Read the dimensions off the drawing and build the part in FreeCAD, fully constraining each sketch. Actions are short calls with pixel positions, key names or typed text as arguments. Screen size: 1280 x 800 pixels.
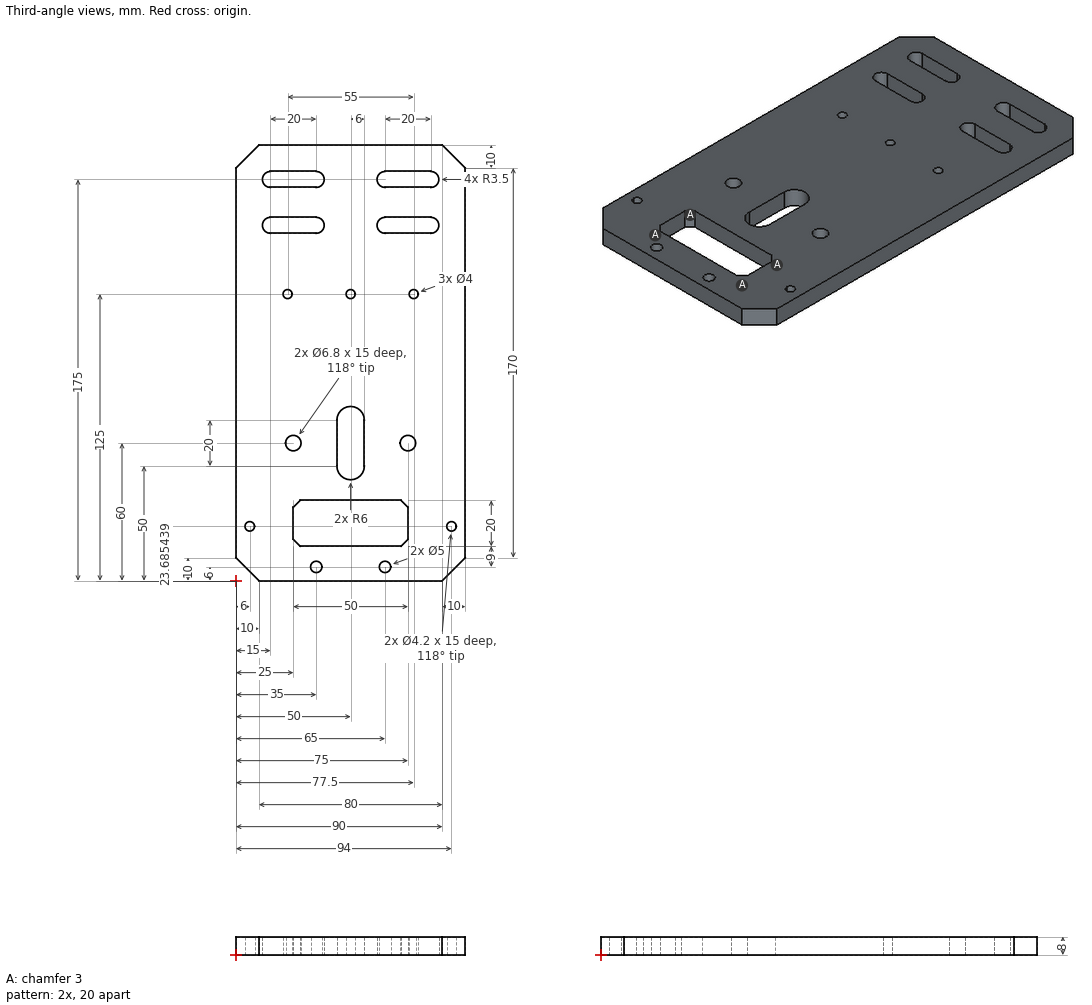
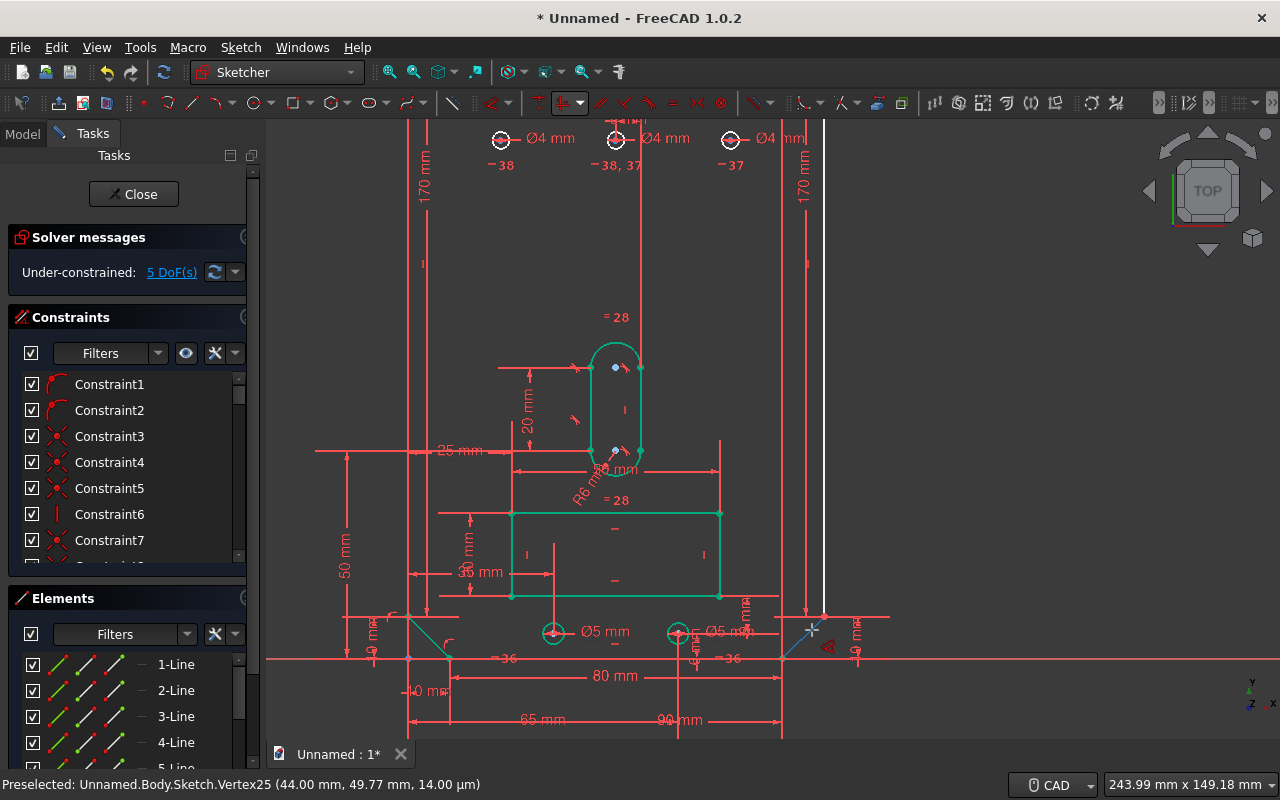
click(812, 629)
click(803, 693)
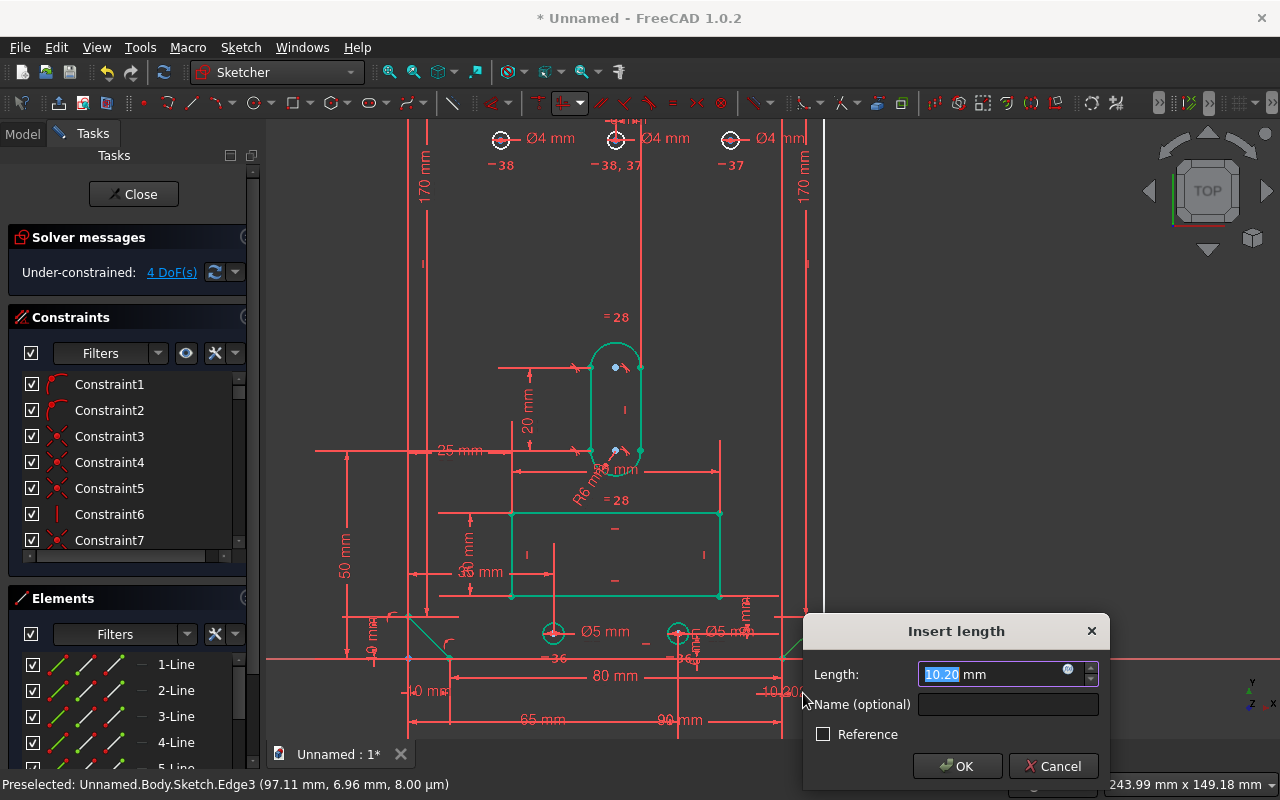
text(10)
key(Return)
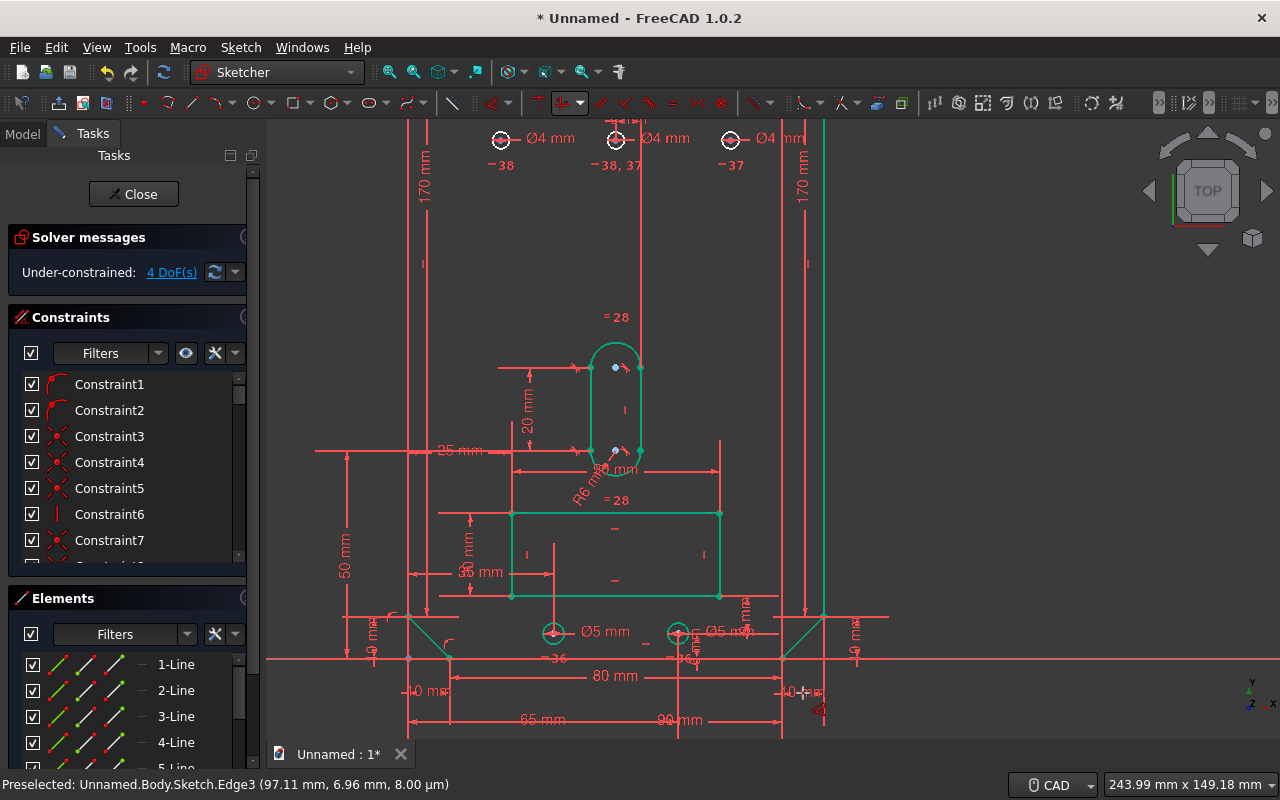
scroll(812, 630, down, 3)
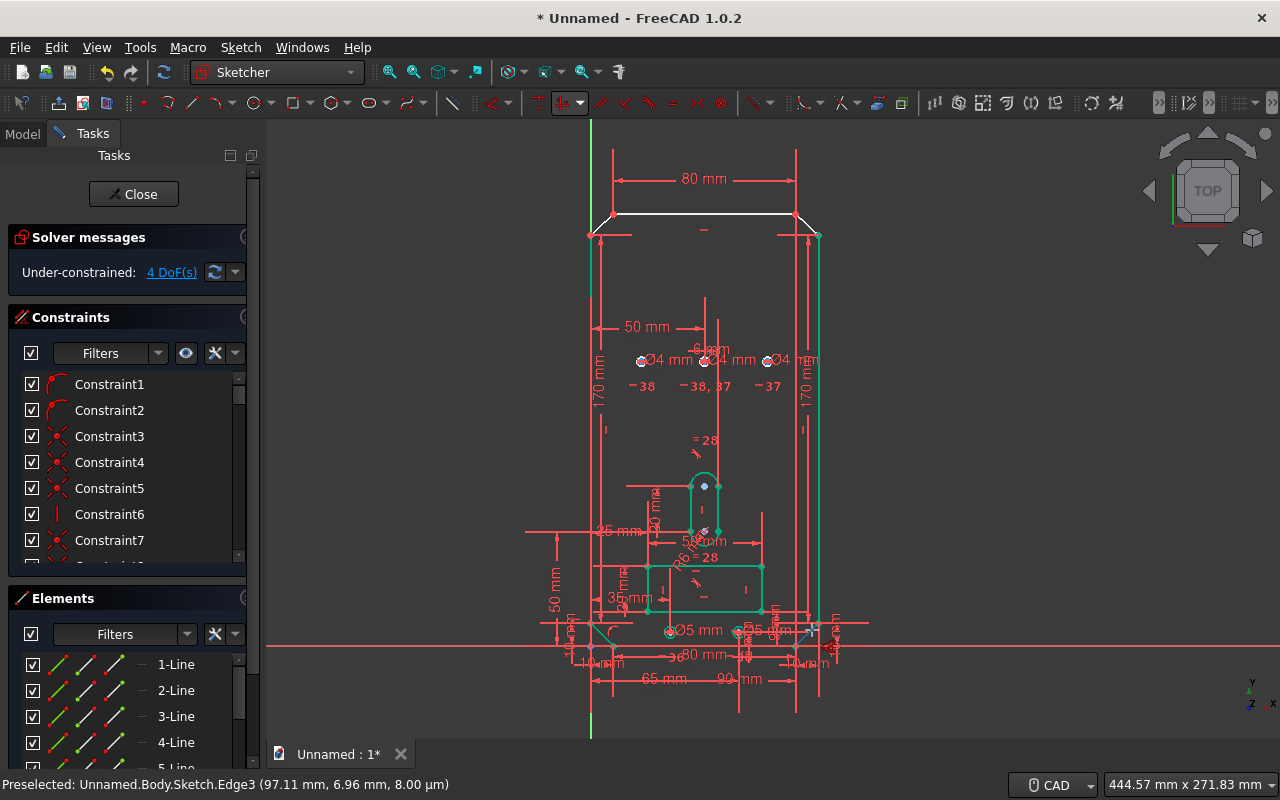
scroll(812, 229, up, 3)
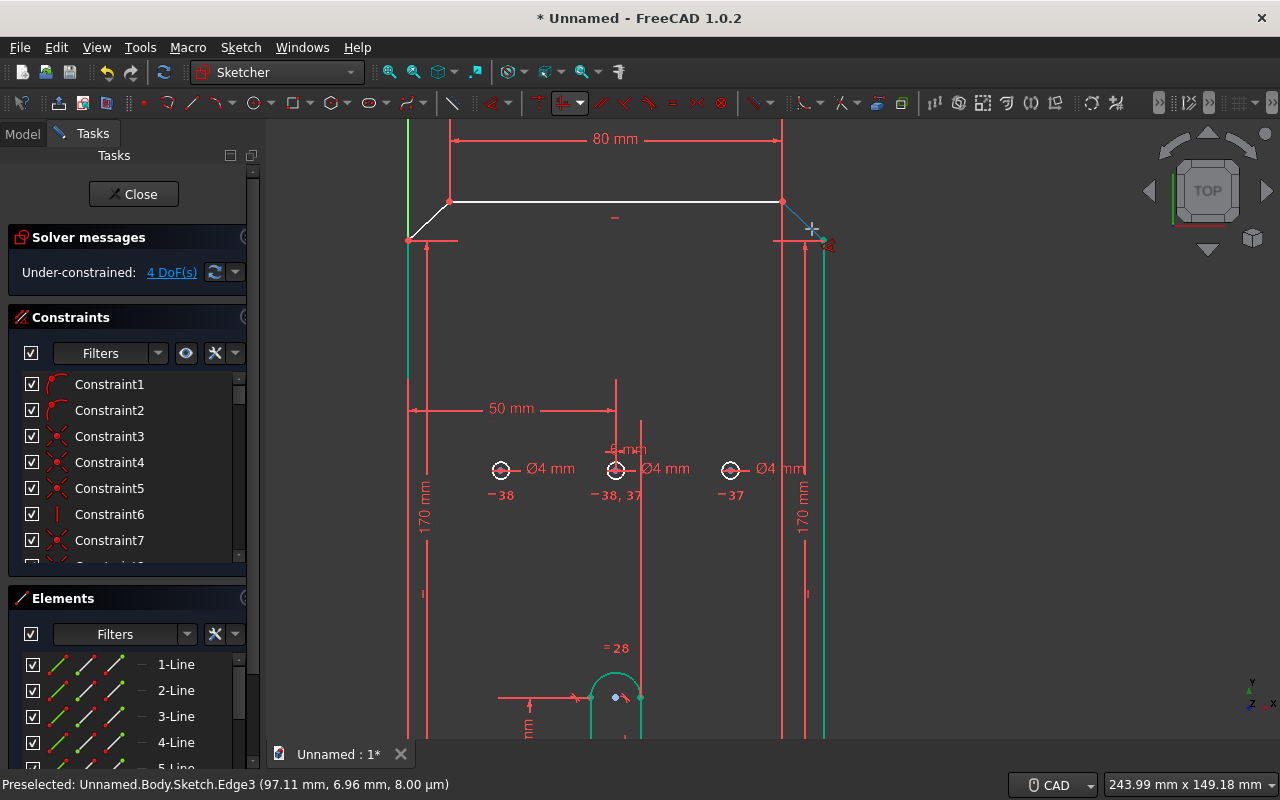
click(811, 229)
click(858, 221)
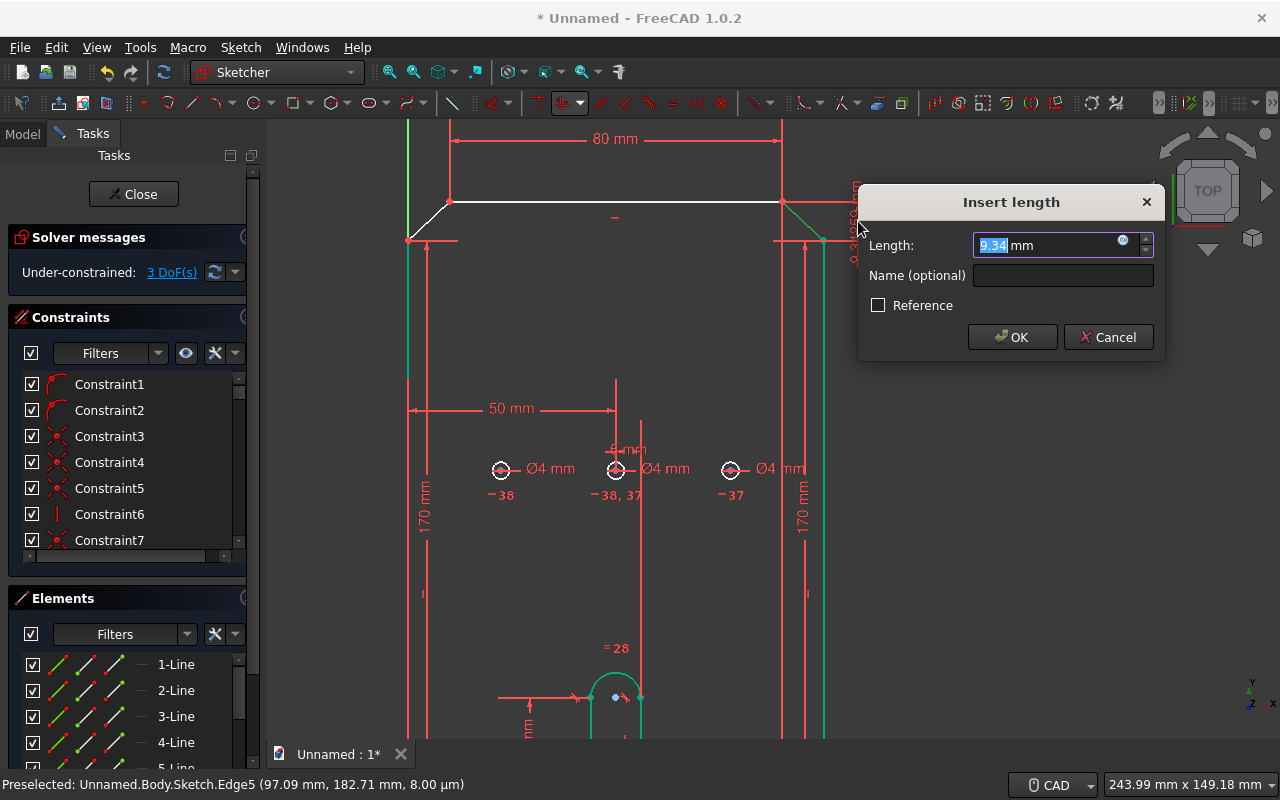
text(10)
key(Return)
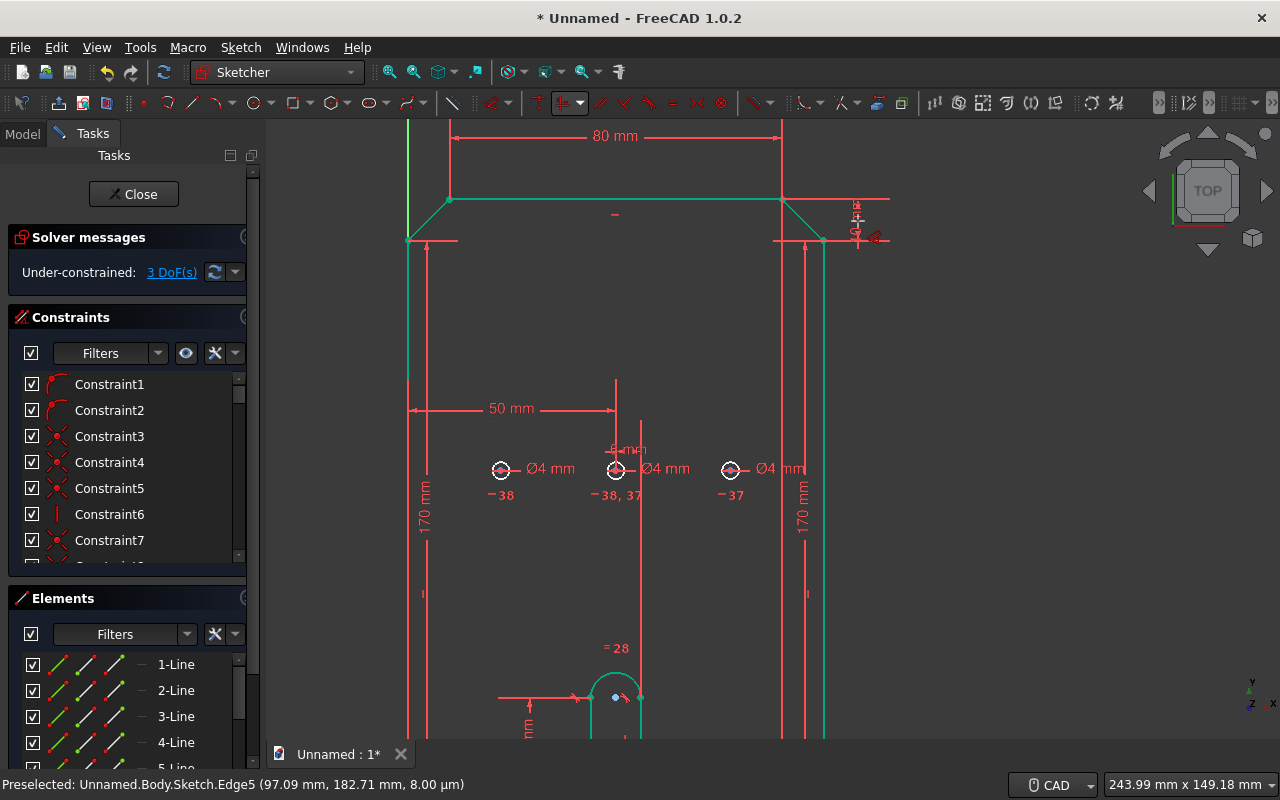
click(731, 471)
click(374, 591)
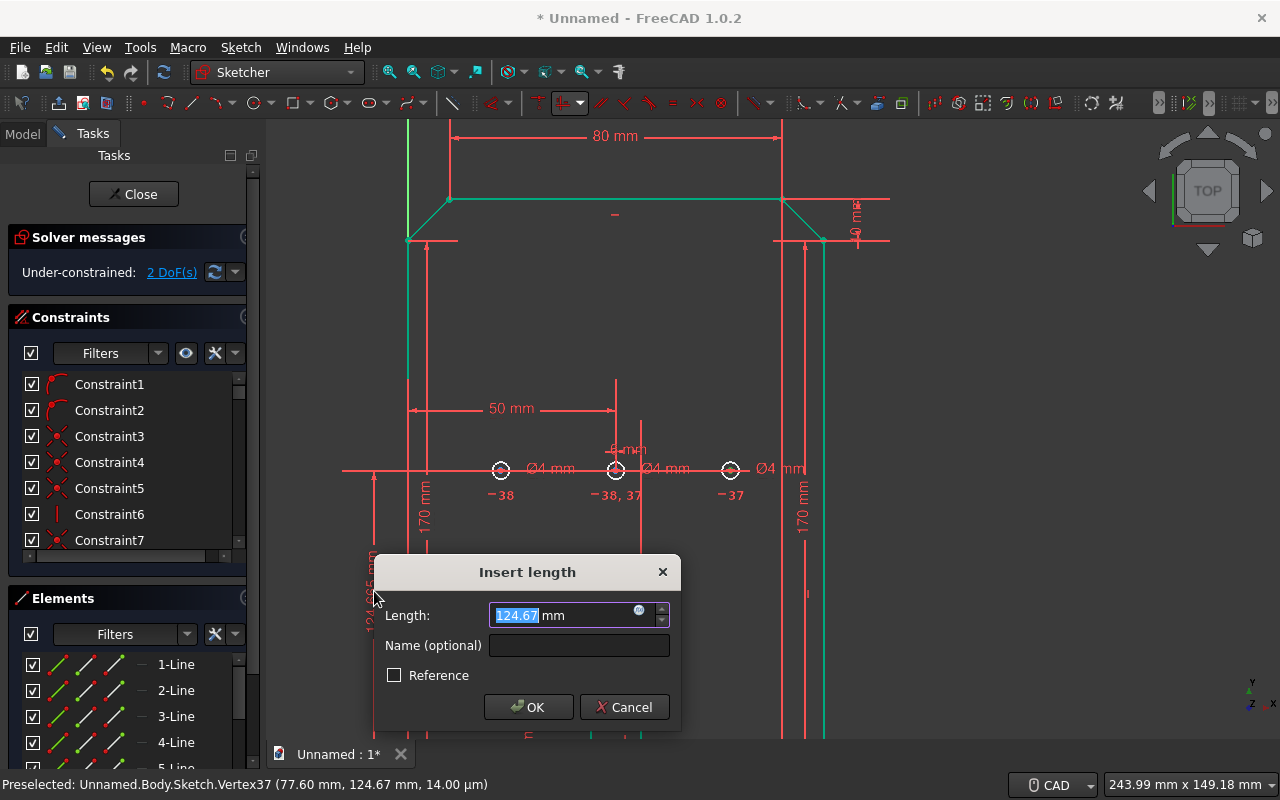
text(125)
key(Return)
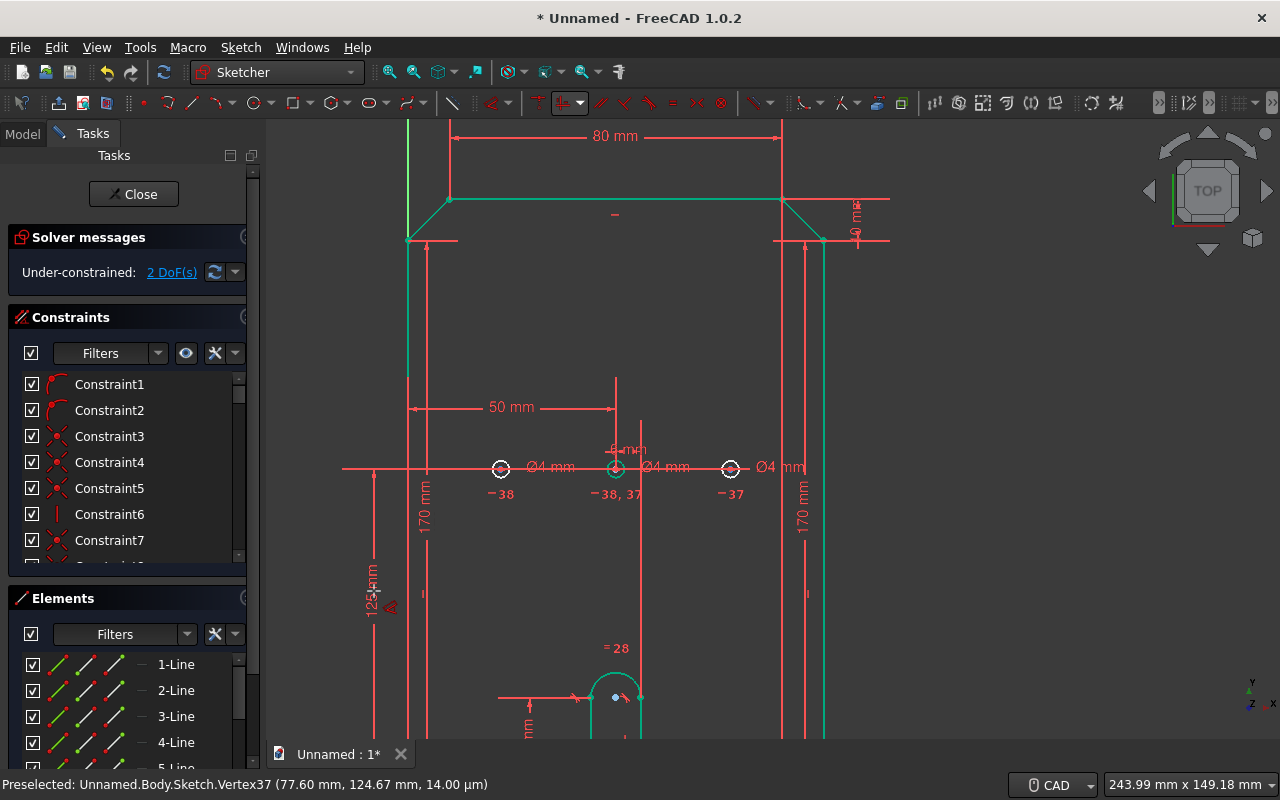
click(731, 469)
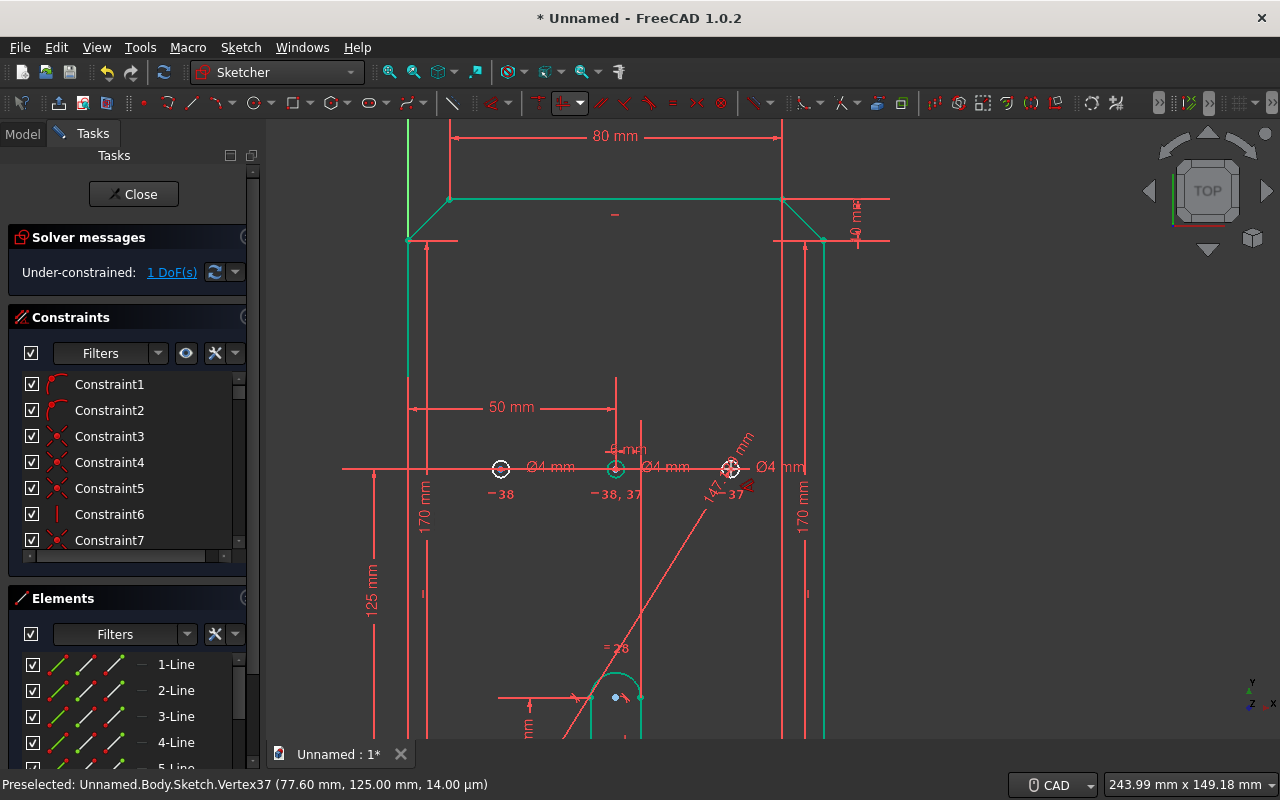
click(501, 469)
click(535, 435)